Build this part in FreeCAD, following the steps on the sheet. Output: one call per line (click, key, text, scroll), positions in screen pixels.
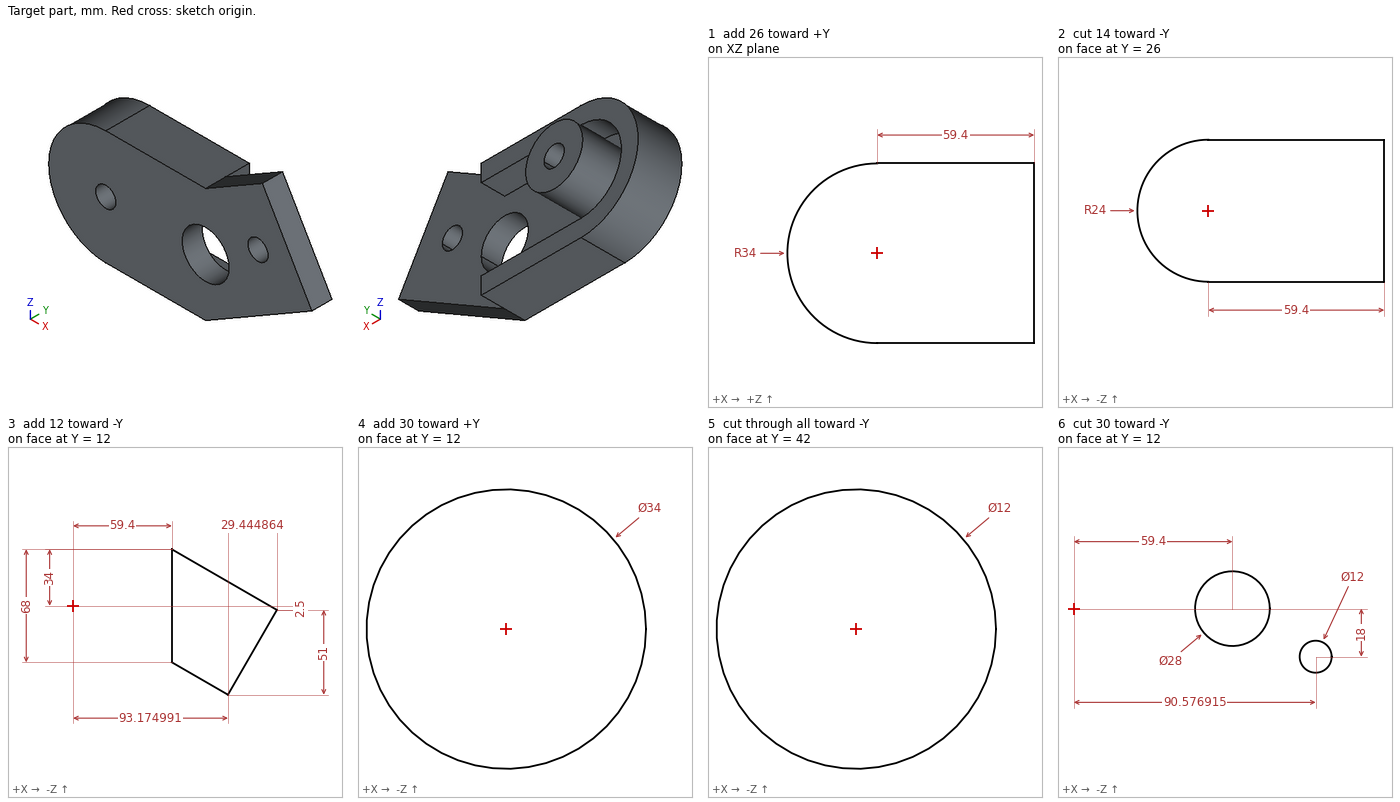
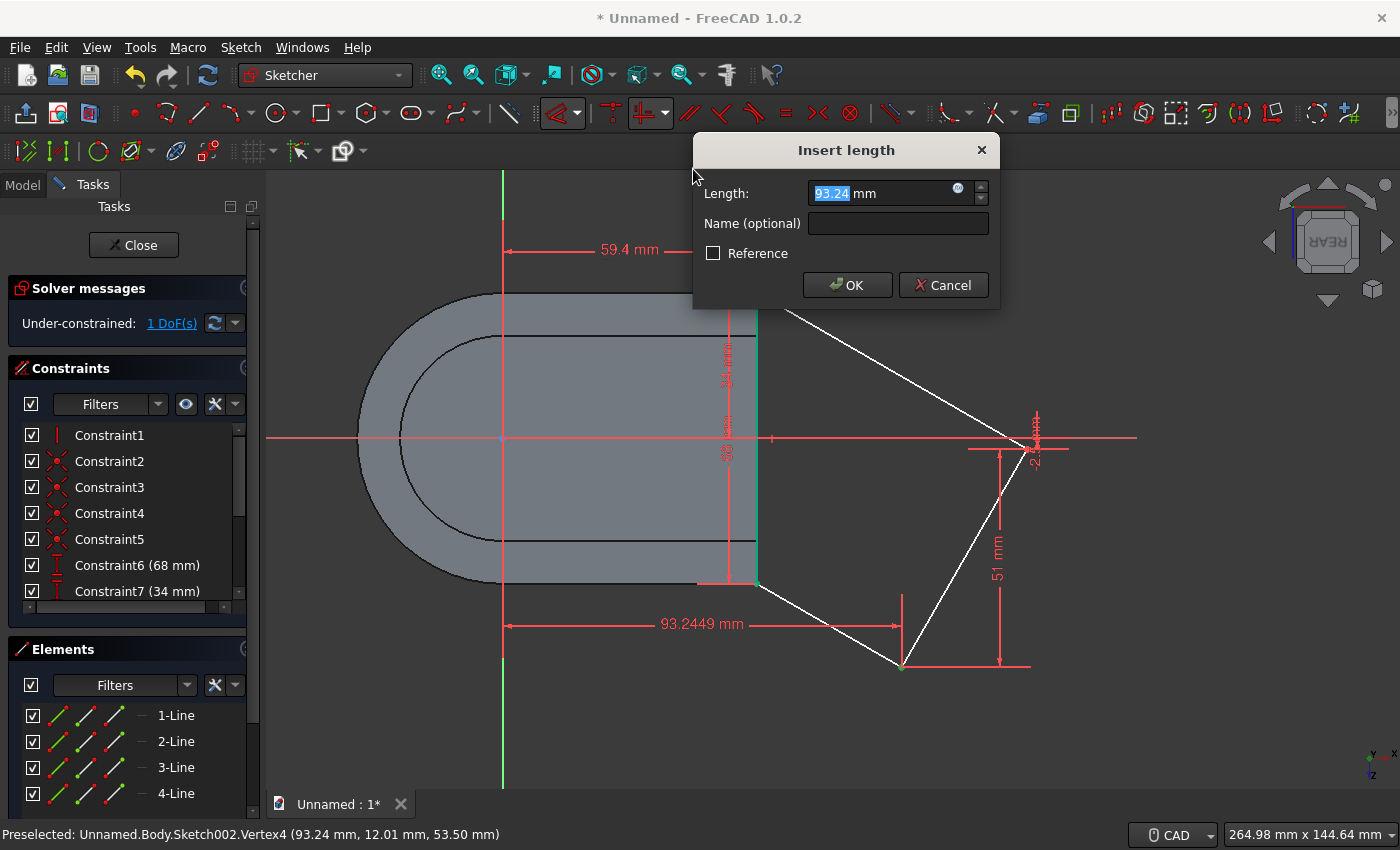
text(93.174991)
key(Return)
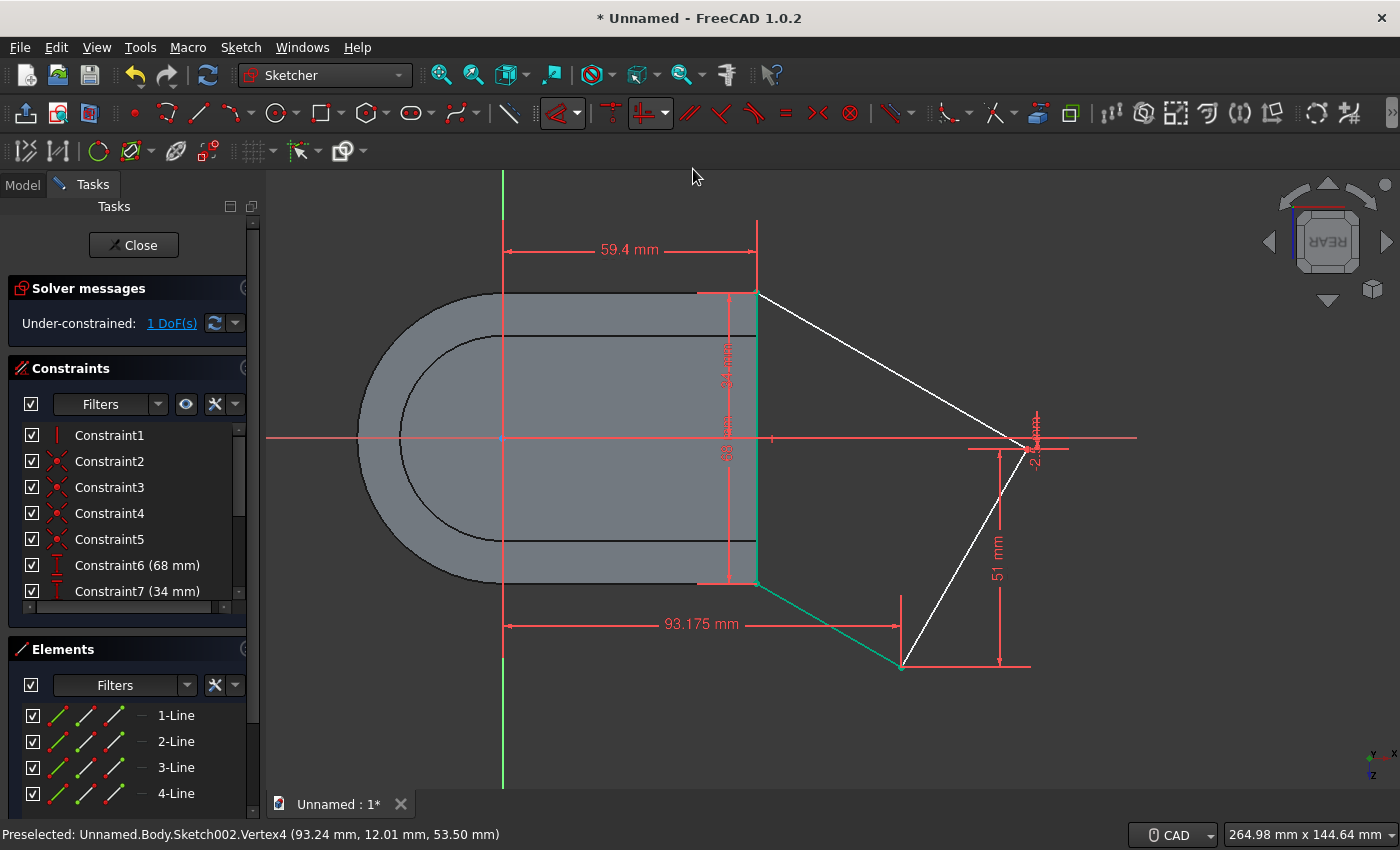
click(939, 602)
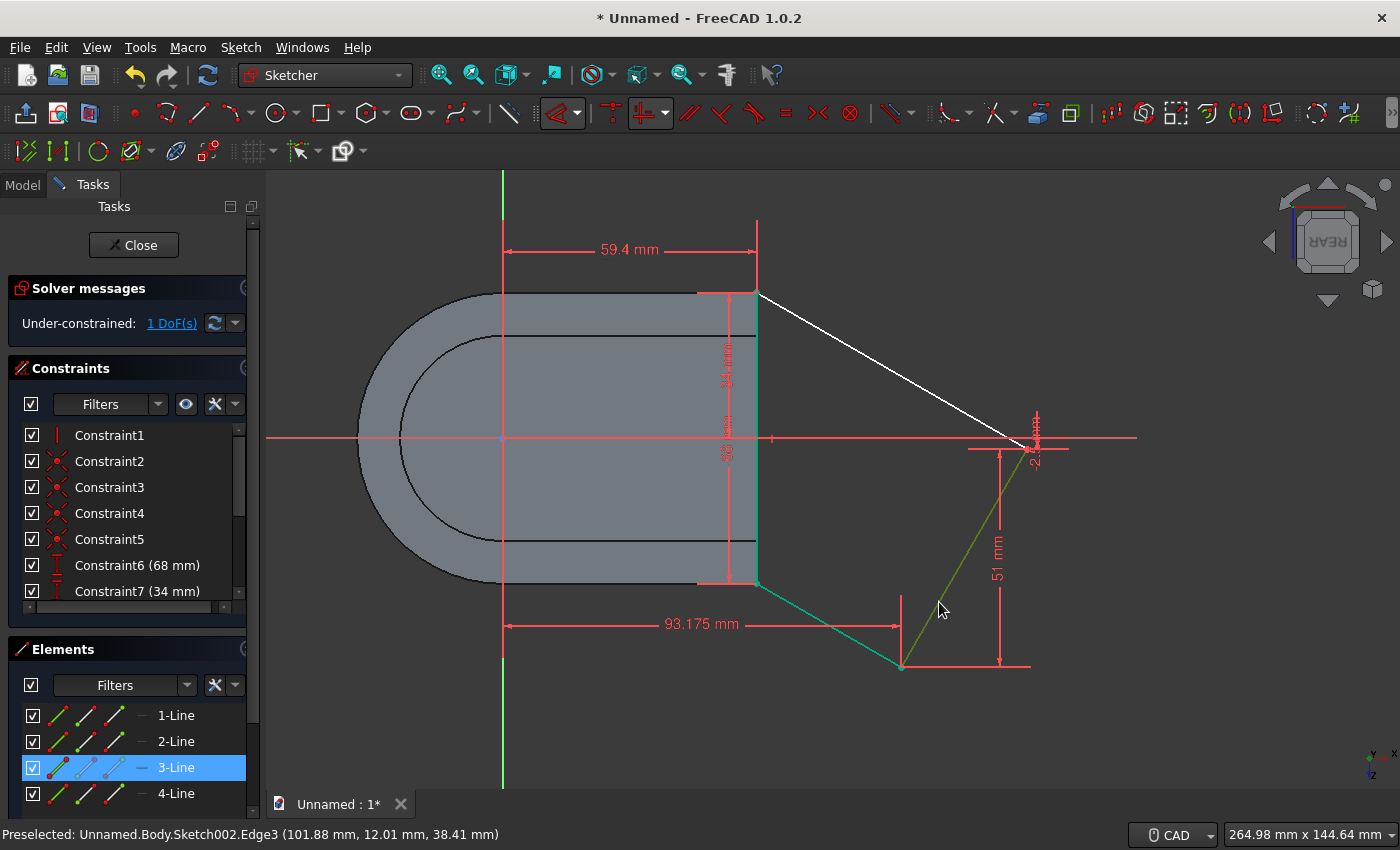
click(580, 114)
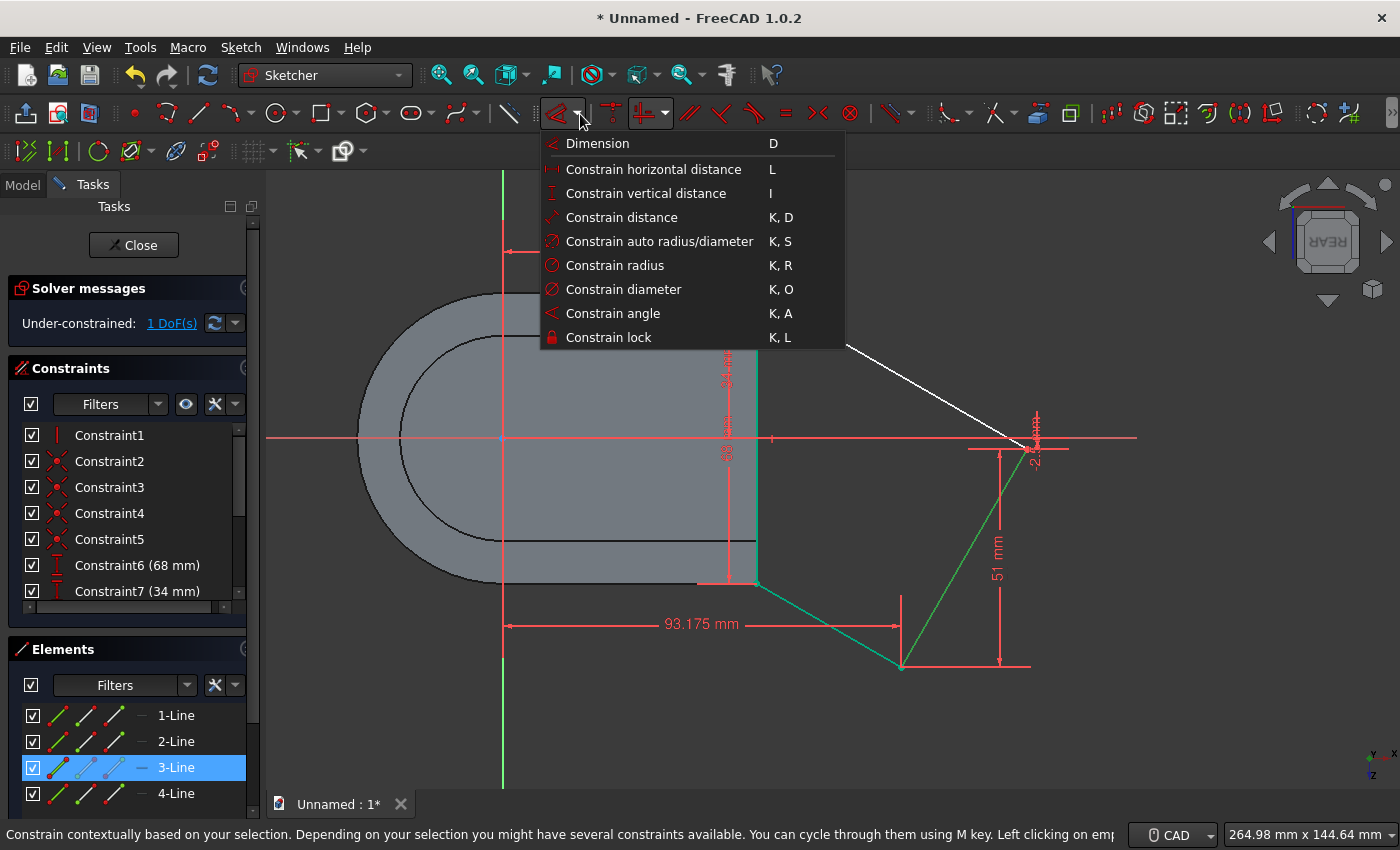
click(693, 169)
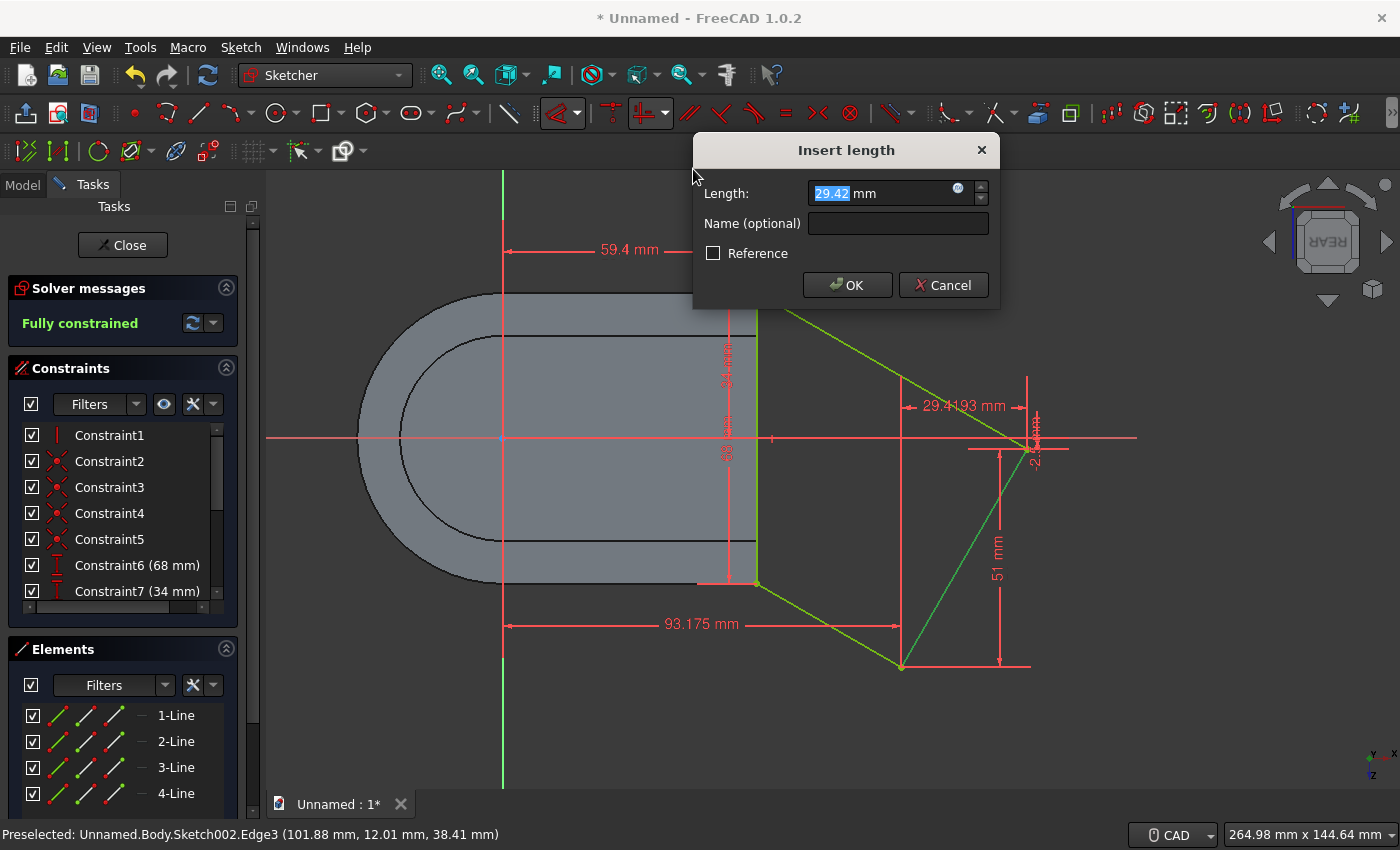
text(29.444864)
key(Return)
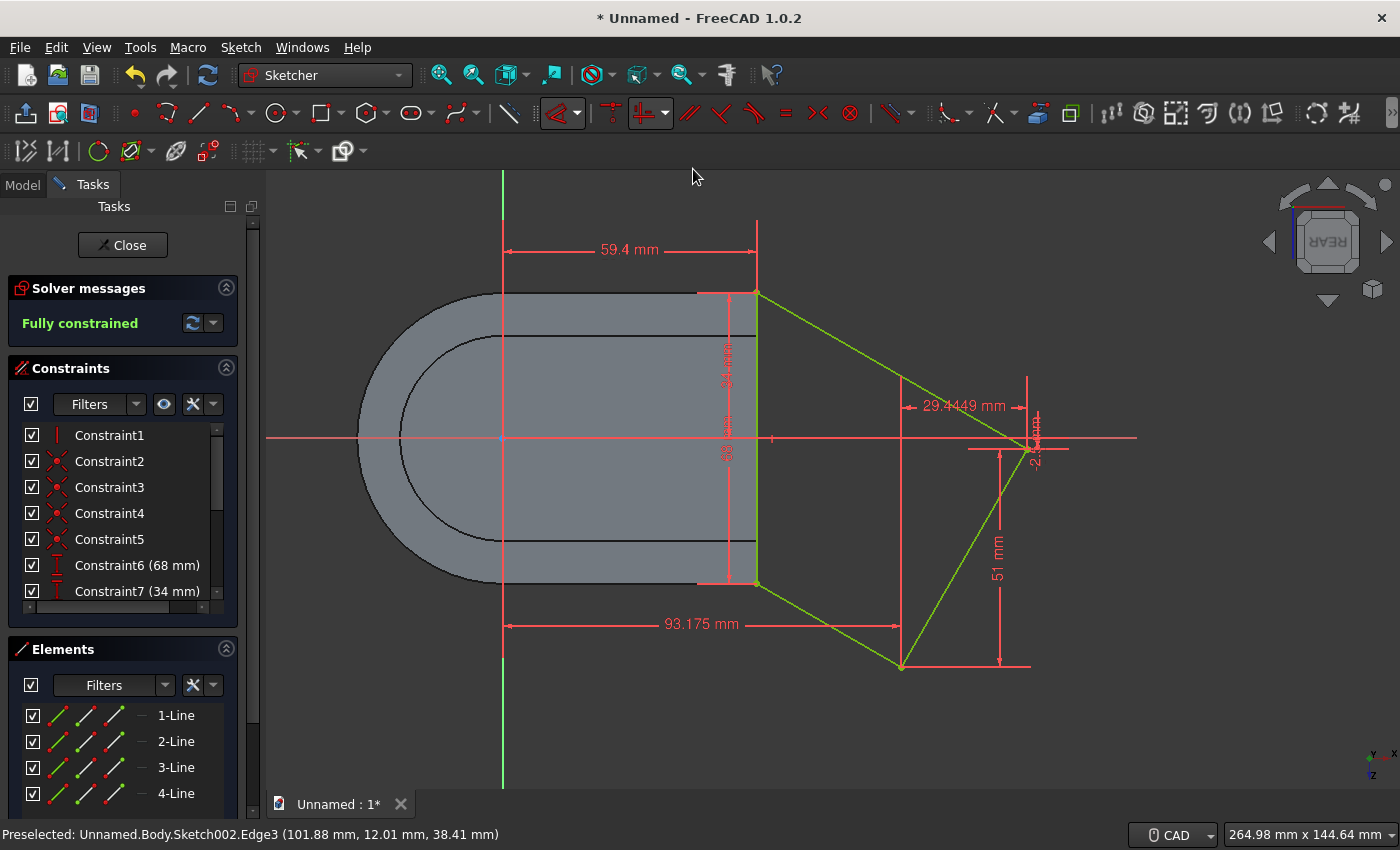
click(123, 245)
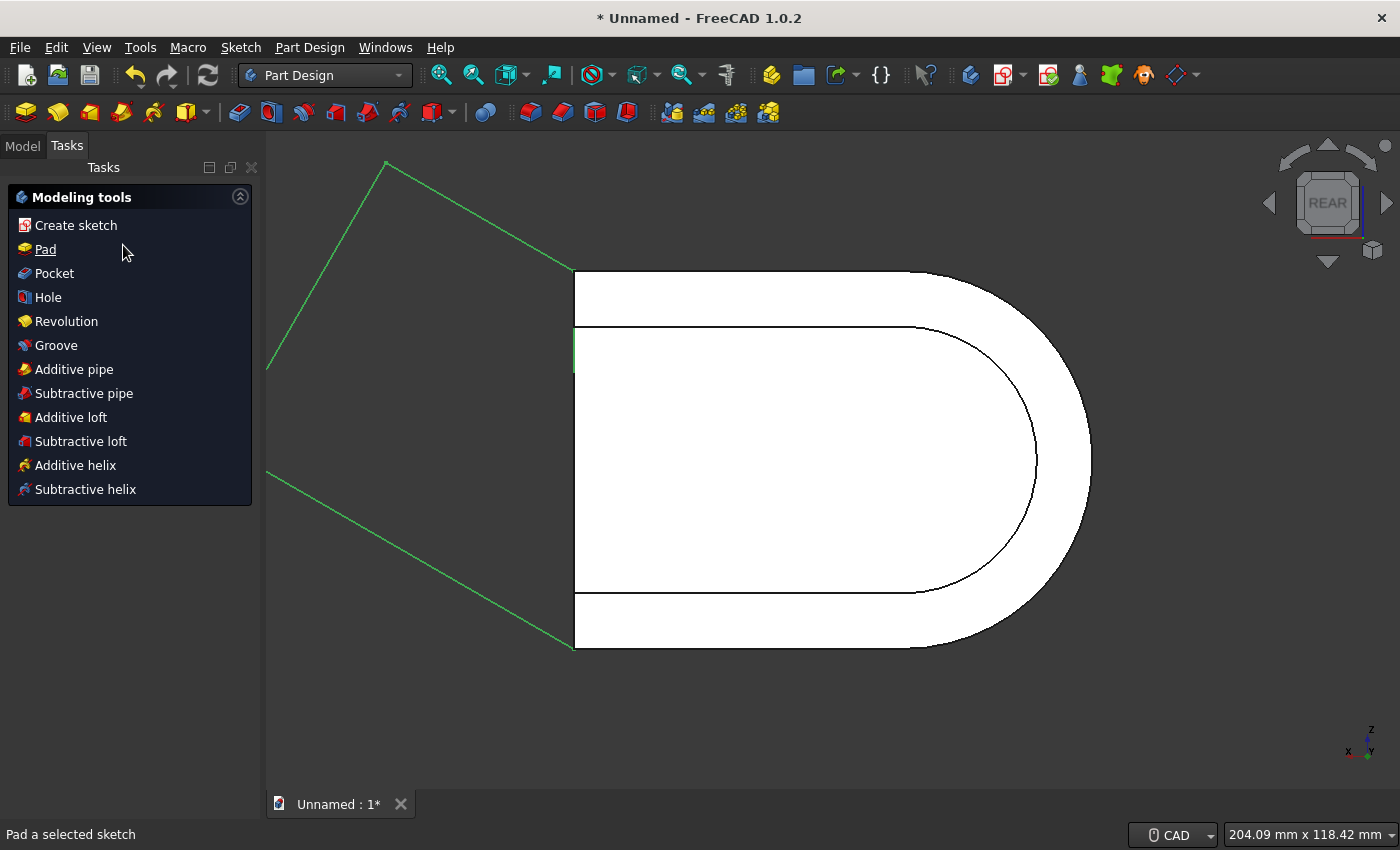
click(26, 112)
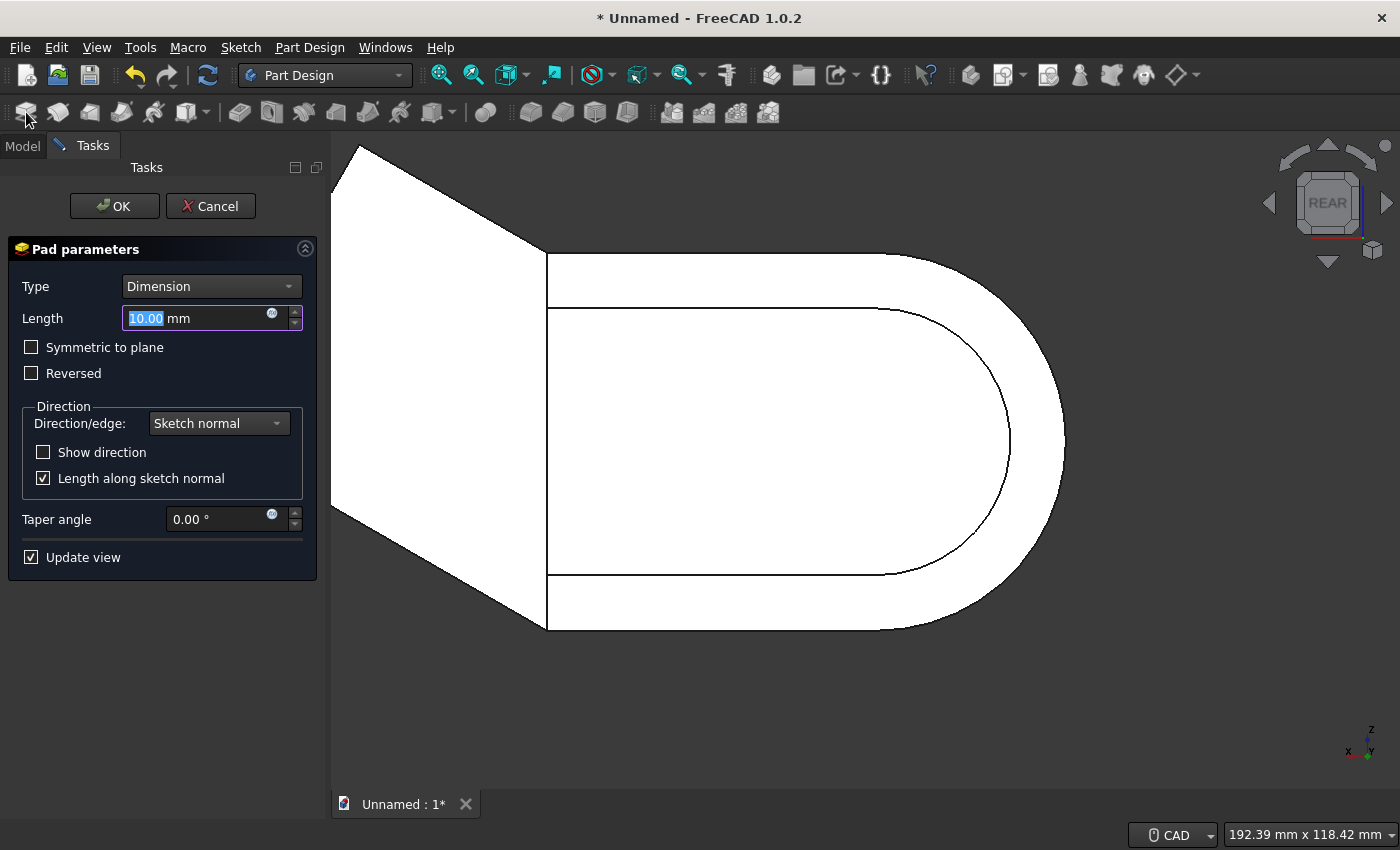
text(12)
key(Tab)